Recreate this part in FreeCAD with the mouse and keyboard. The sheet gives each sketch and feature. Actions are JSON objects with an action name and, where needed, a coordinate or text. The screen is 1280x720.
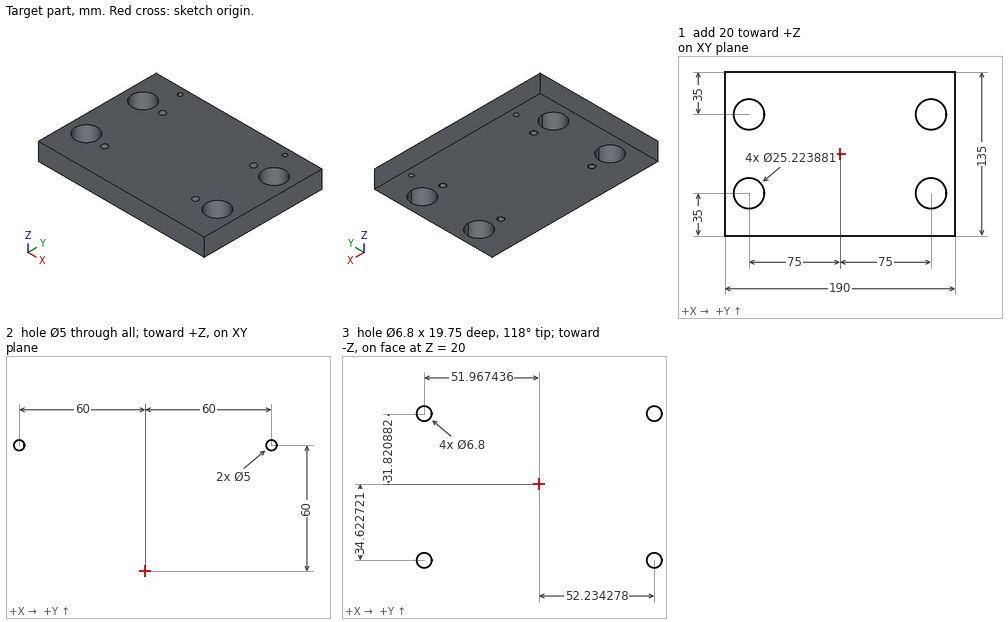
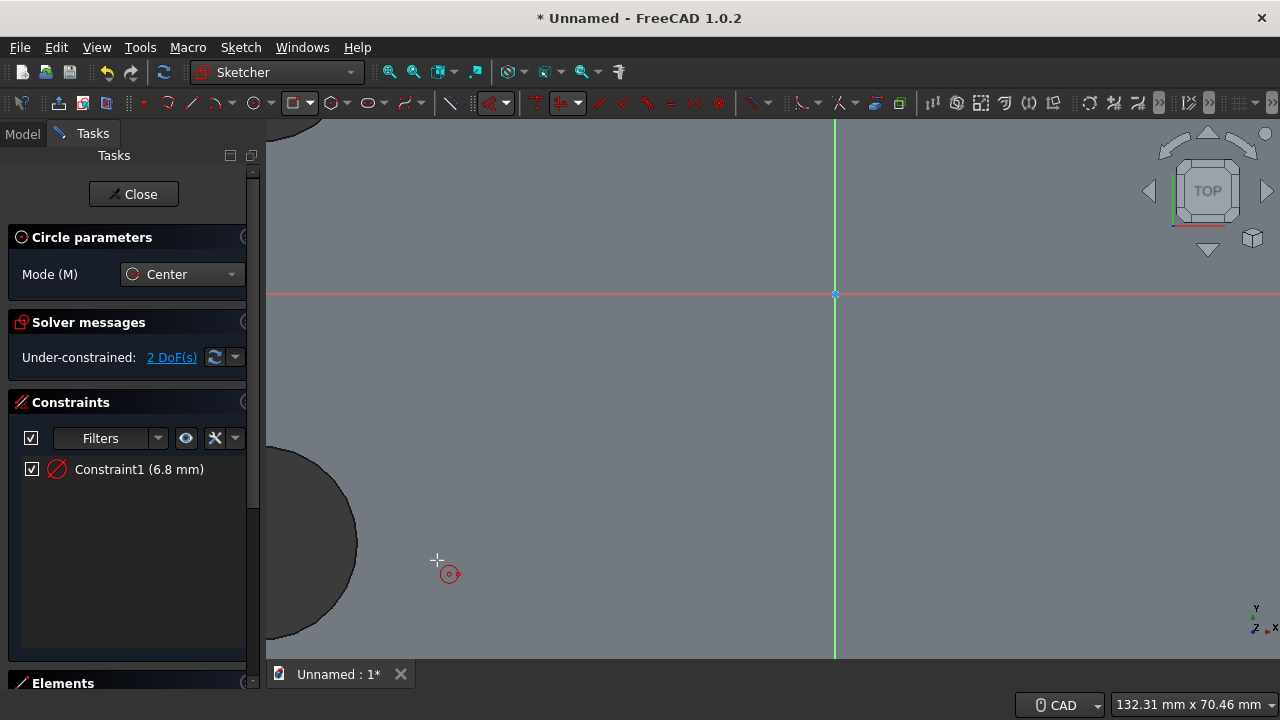
{"action": "left_click", "coordinate": [437, 559]}
{"action": "mouse_move", "coordinate": [455, 541]}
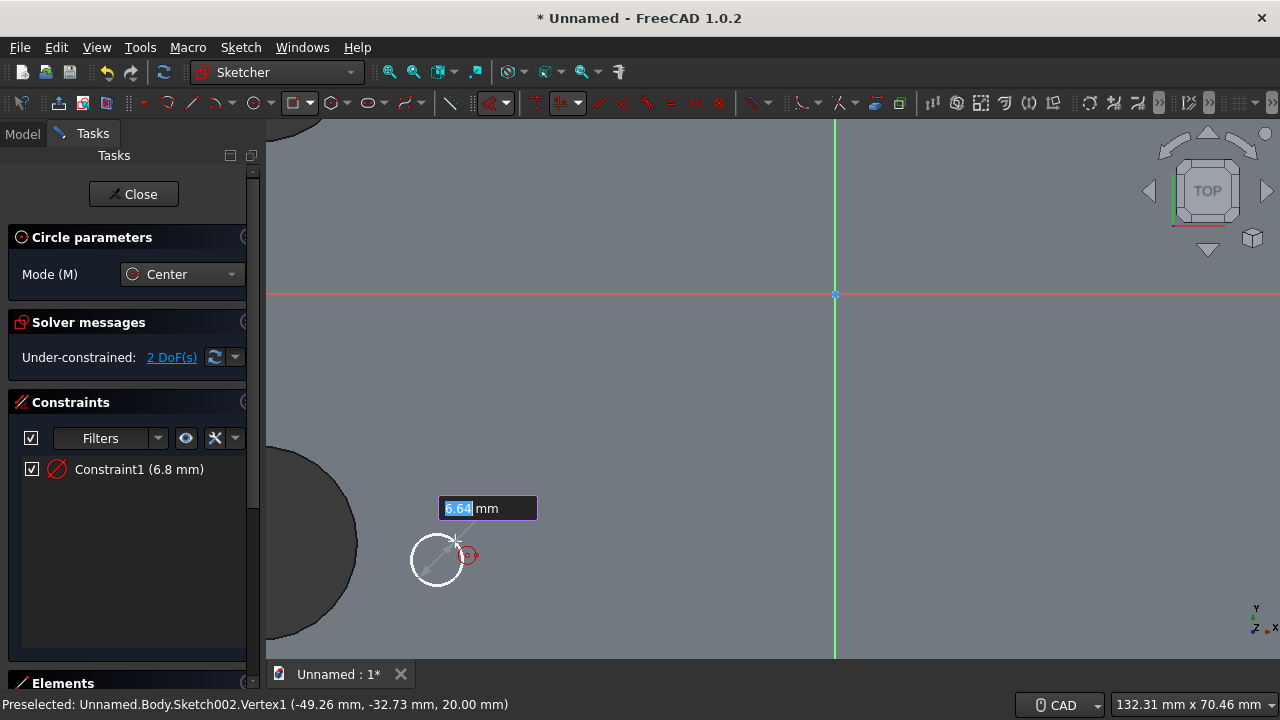
{"action": "type", "text": "6.8"}
{"action": "key", "text": "Return"}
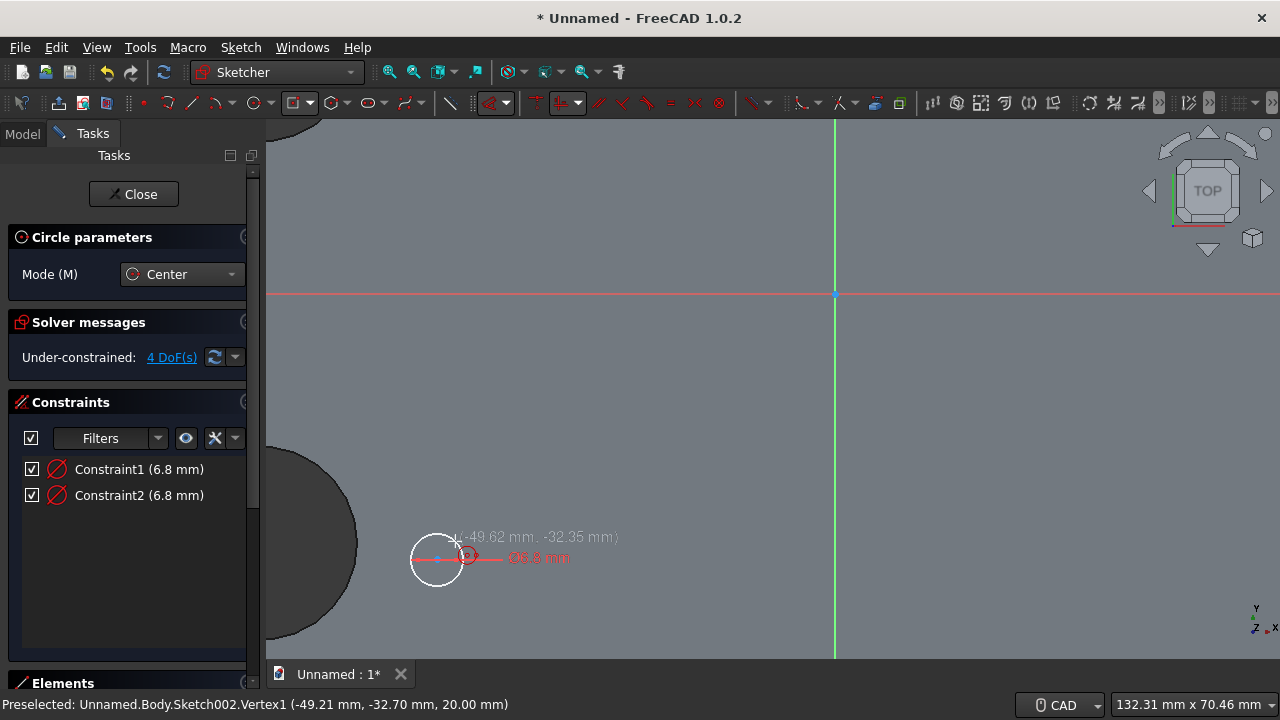
{"action": "scroll", "coordinate": [437, 560], "scroll_direction": "down", "scroll_amount": 2}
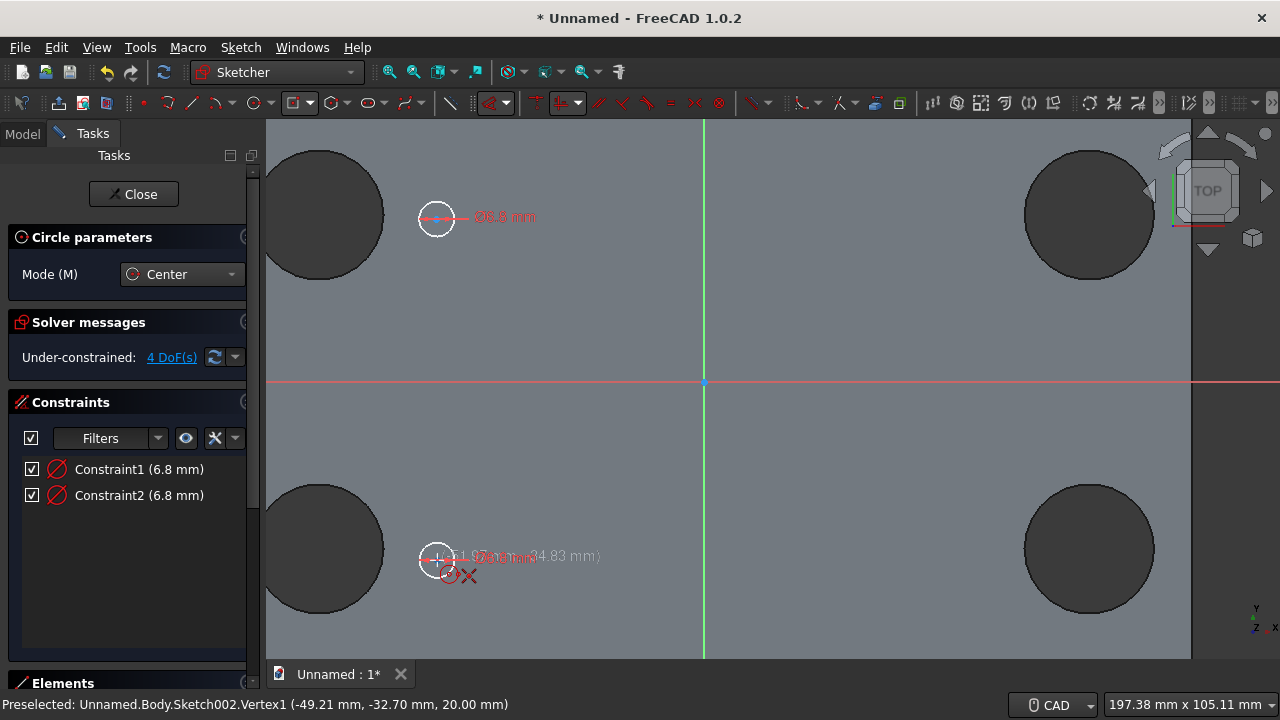
{"action": "scroll", "coordinate": [972, 560], "scroll_direction": "up", "scroll_amount": 2}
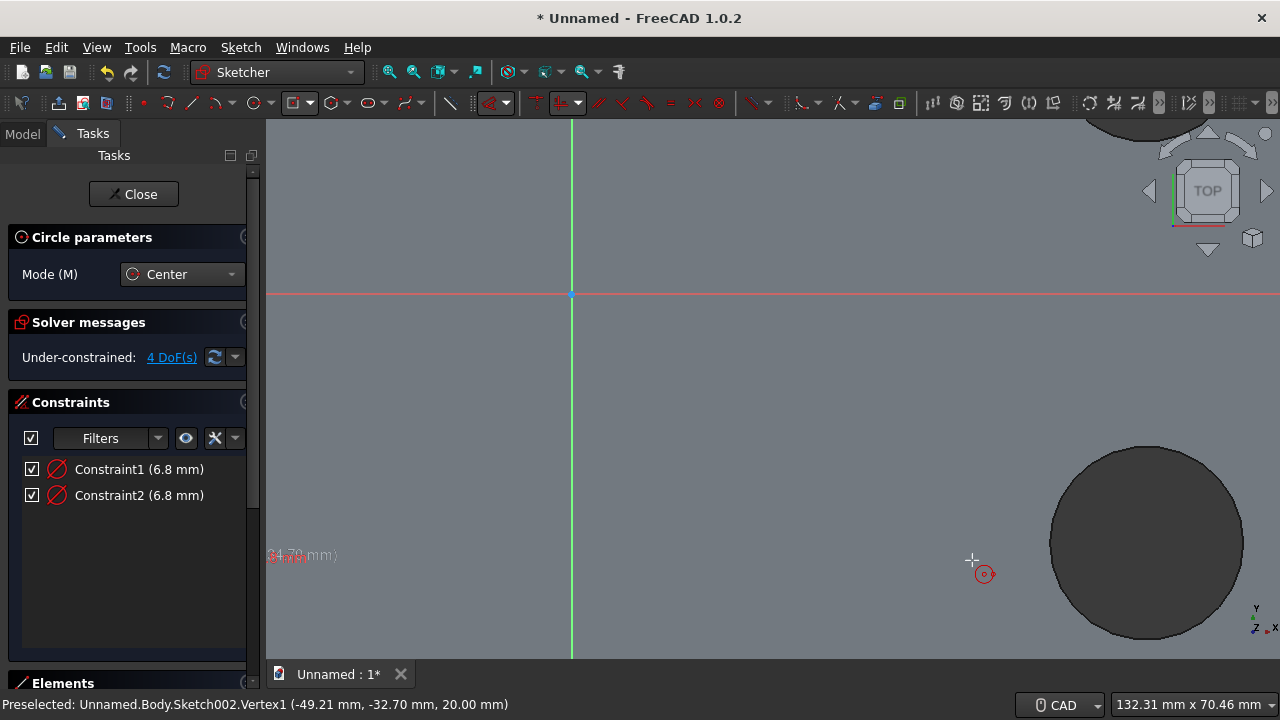
{"action": "left_click", "coordinate": [972, 559]}
{"action": "mouse_move", "coordinate": [991, 541]}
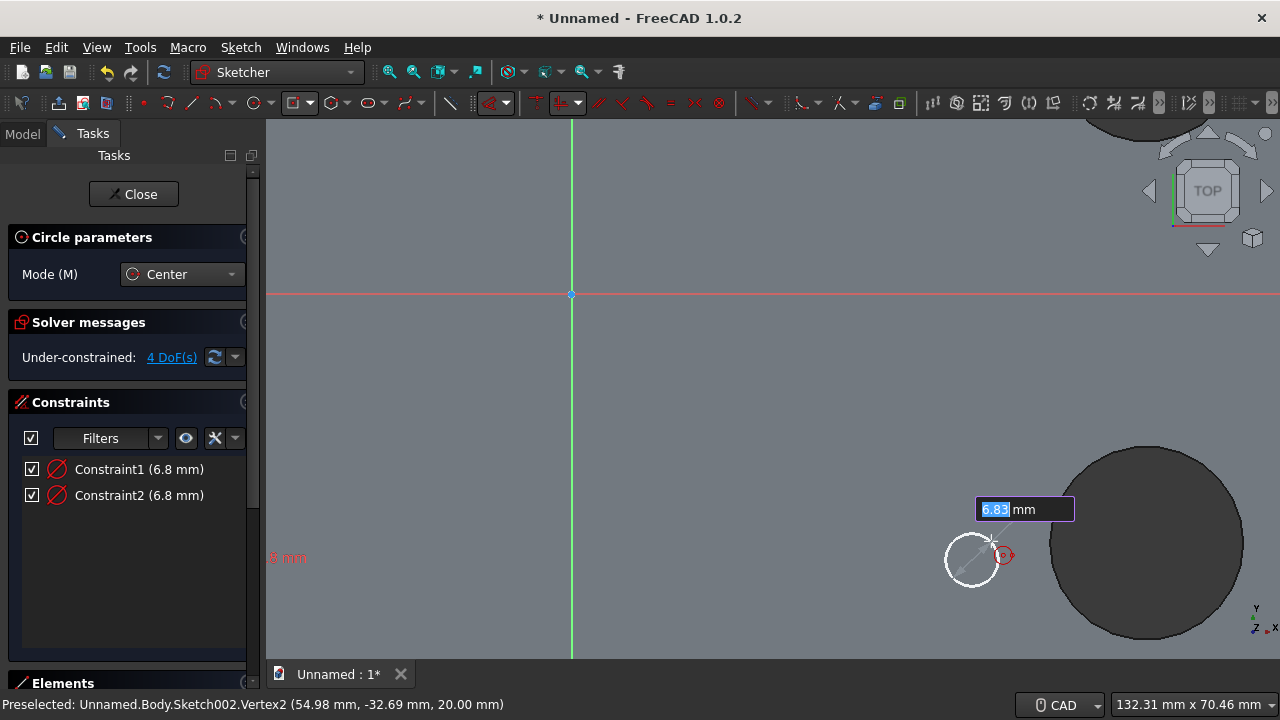
{"action": "type", "text": "6.8"}
{"action": "key", "text": "Return"}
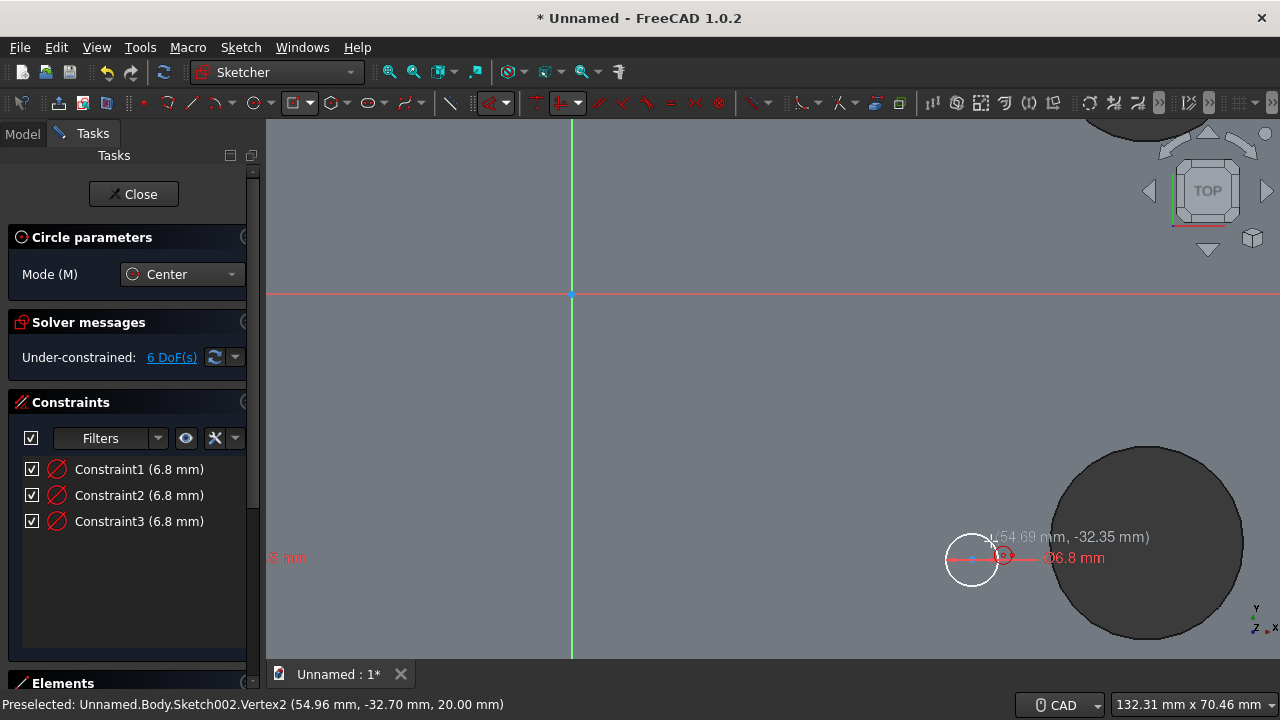
{"action": "scroll", "coordinate": [972, 560], "scroll_direction": "down", "scroll_amount": 2}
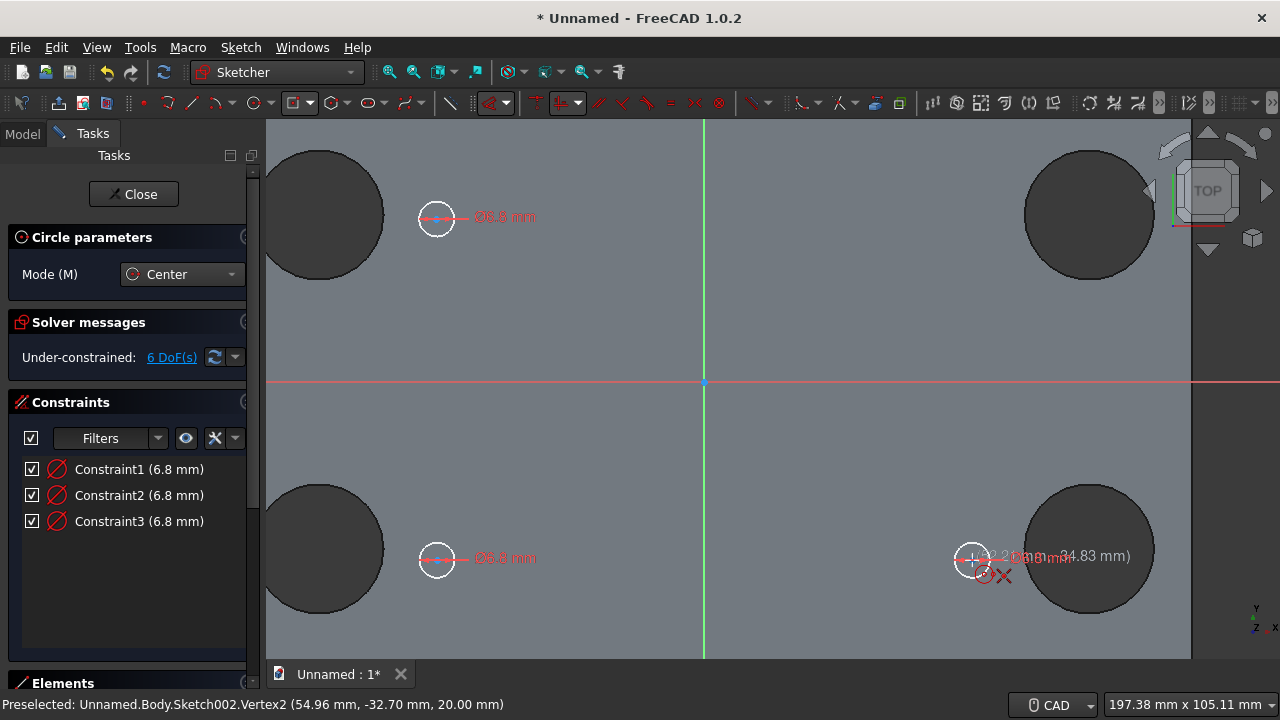
{"action": "scroll", "coordinate": [972, 219], "scroll_direction": "up", "scroll_amount": 2}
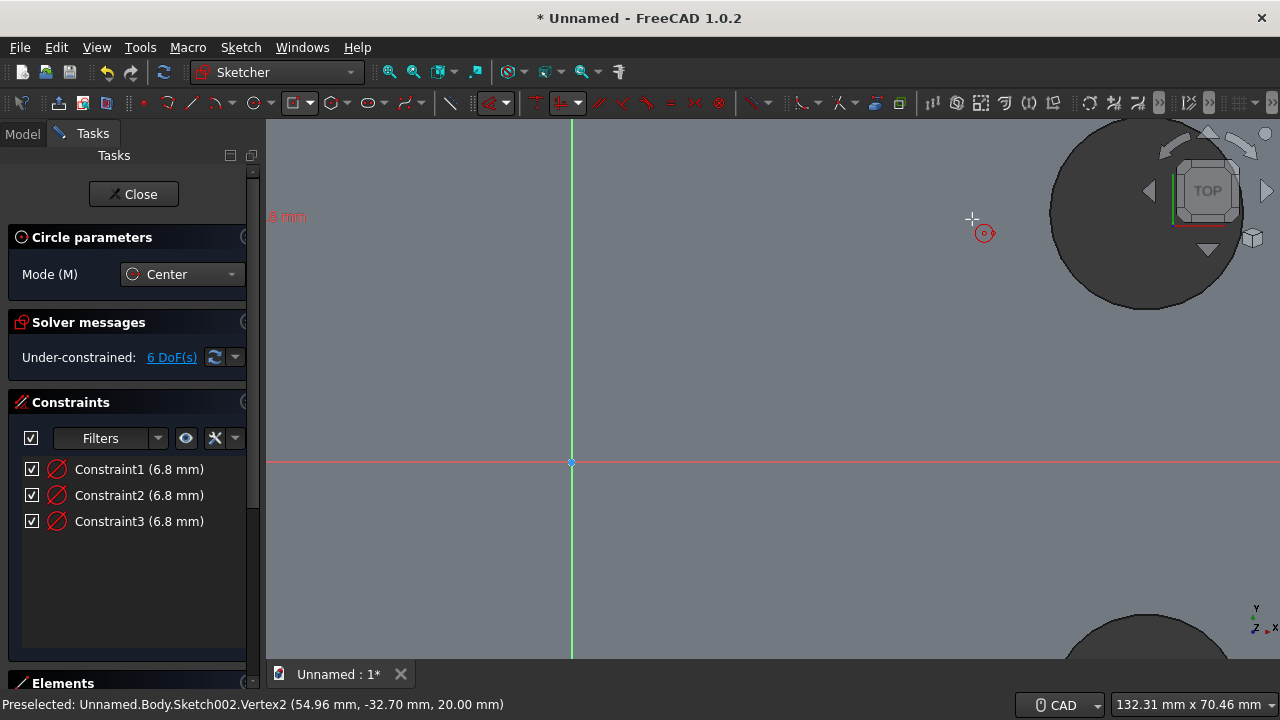
{"action": "left_click", "coordinate": [972, 218]}
{"action": "mouse_move", "coordinate": [991, 200]}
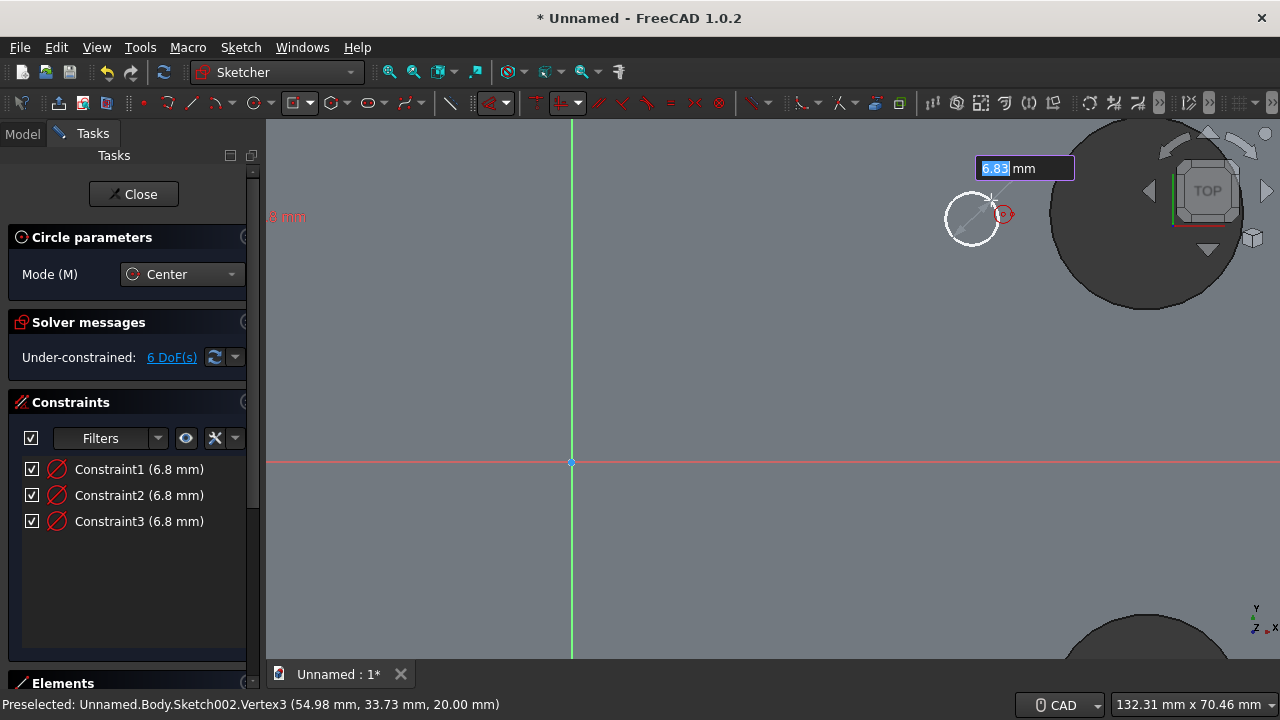
{"action": "type", "text": "6.8"}
{"action": "key", "text": "Return"}
{"action": "key", "text": "Escape"}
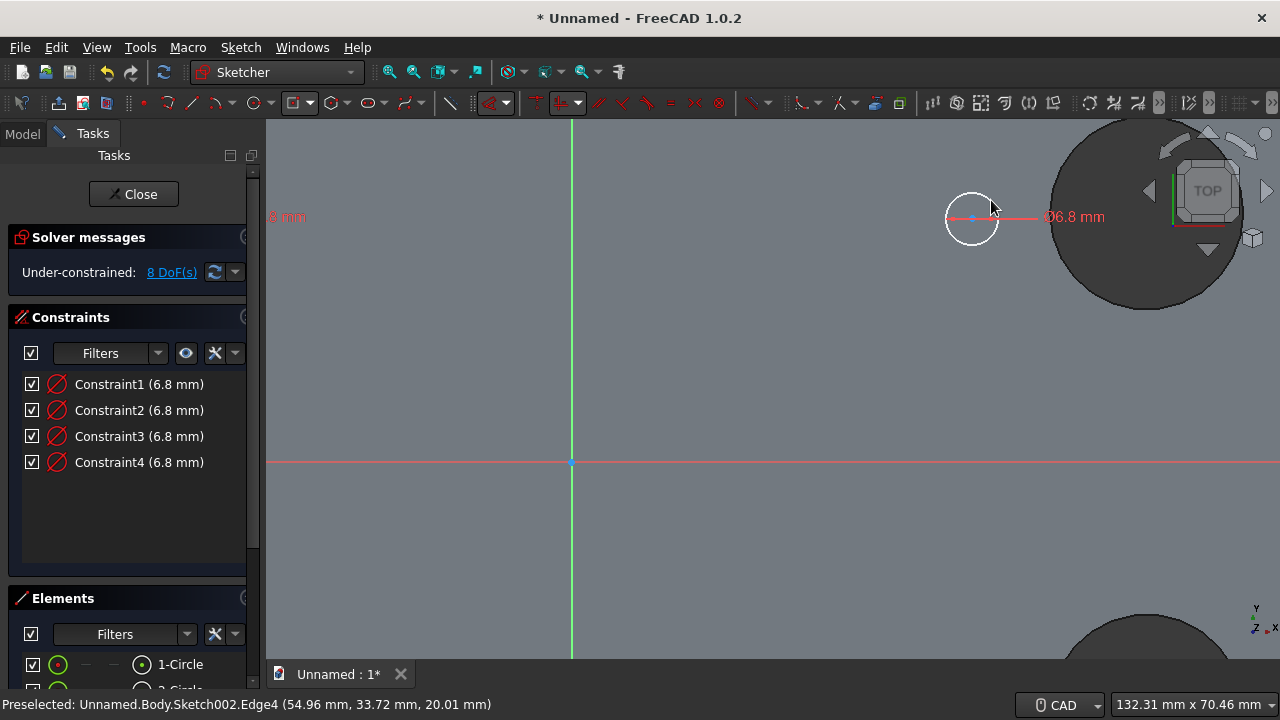
{"action": "scroll", "coordinate": [972, 219], "scroll_direction": "down", "scroll_amount": 2}